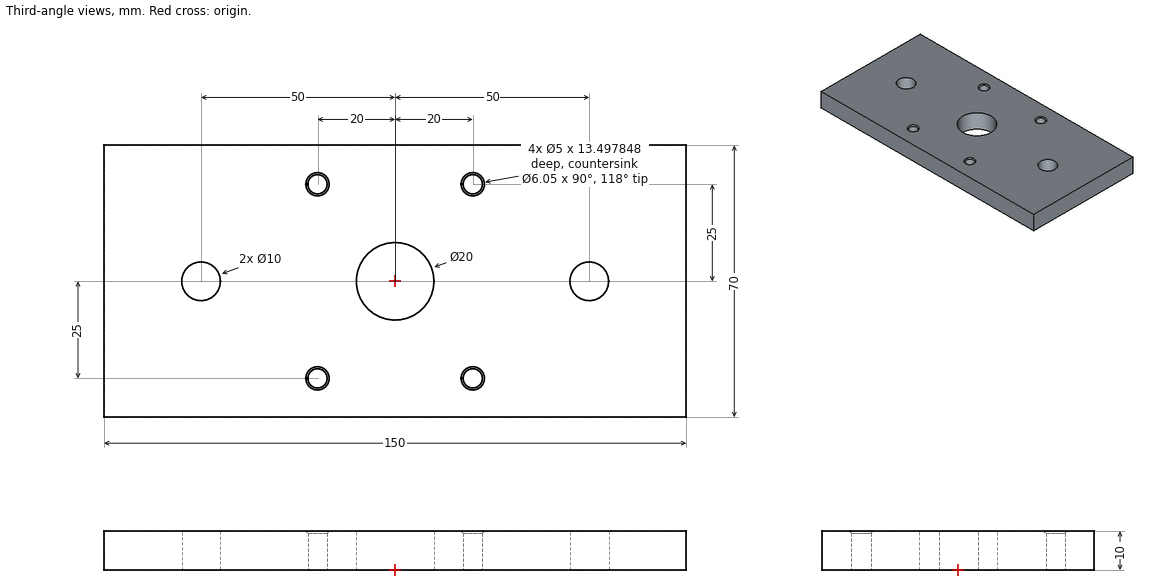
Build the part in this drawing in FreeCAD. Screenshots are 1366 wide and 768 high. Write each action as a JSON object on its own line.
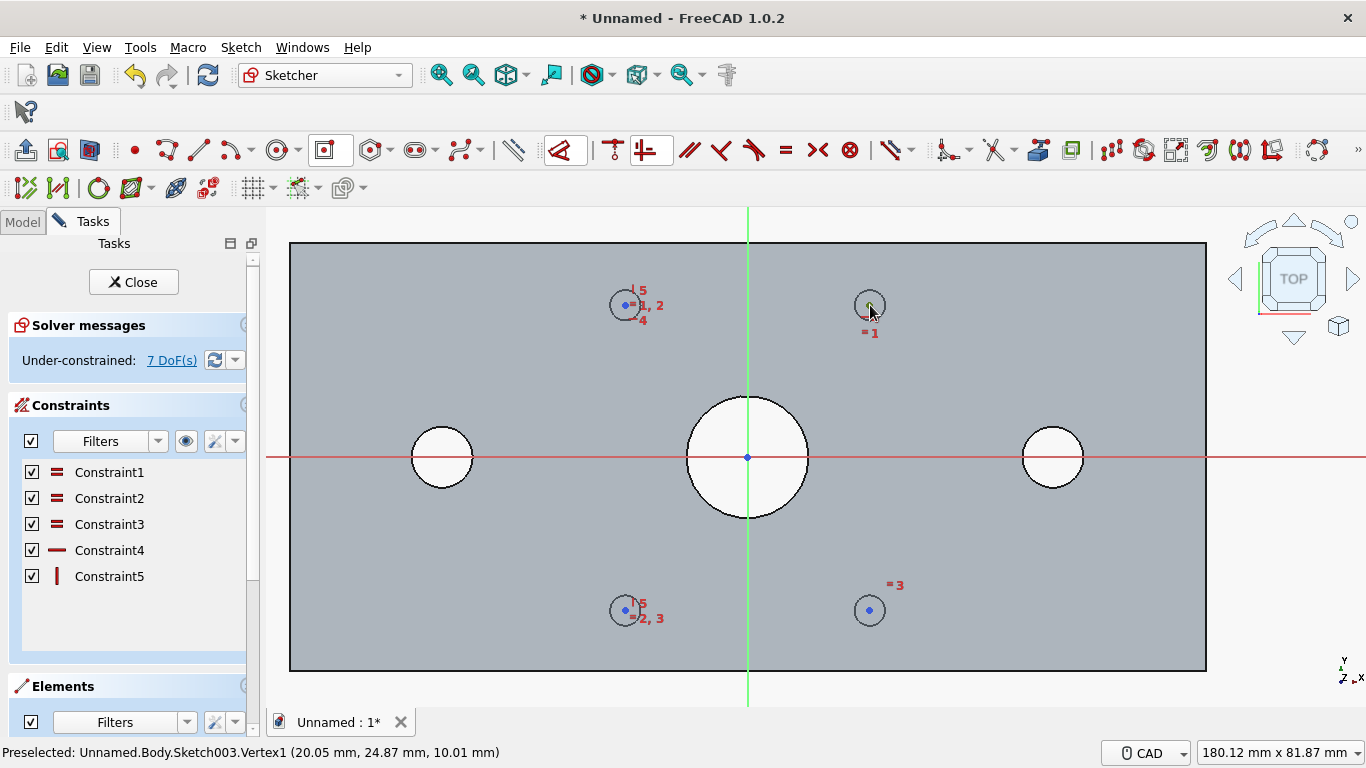
{"action": "left_click", "coordinate": [870, 611]}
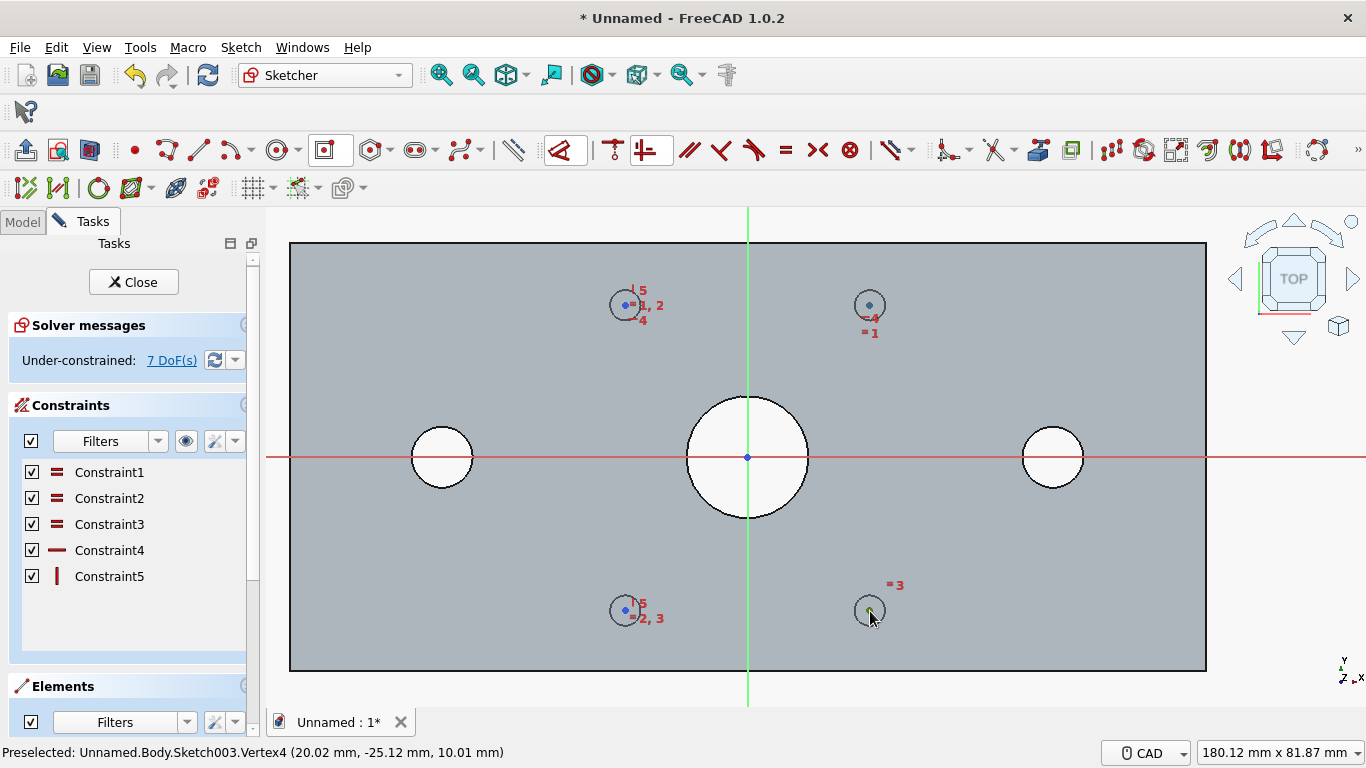
{"action": "left_click", "coordinate": [668, 150]}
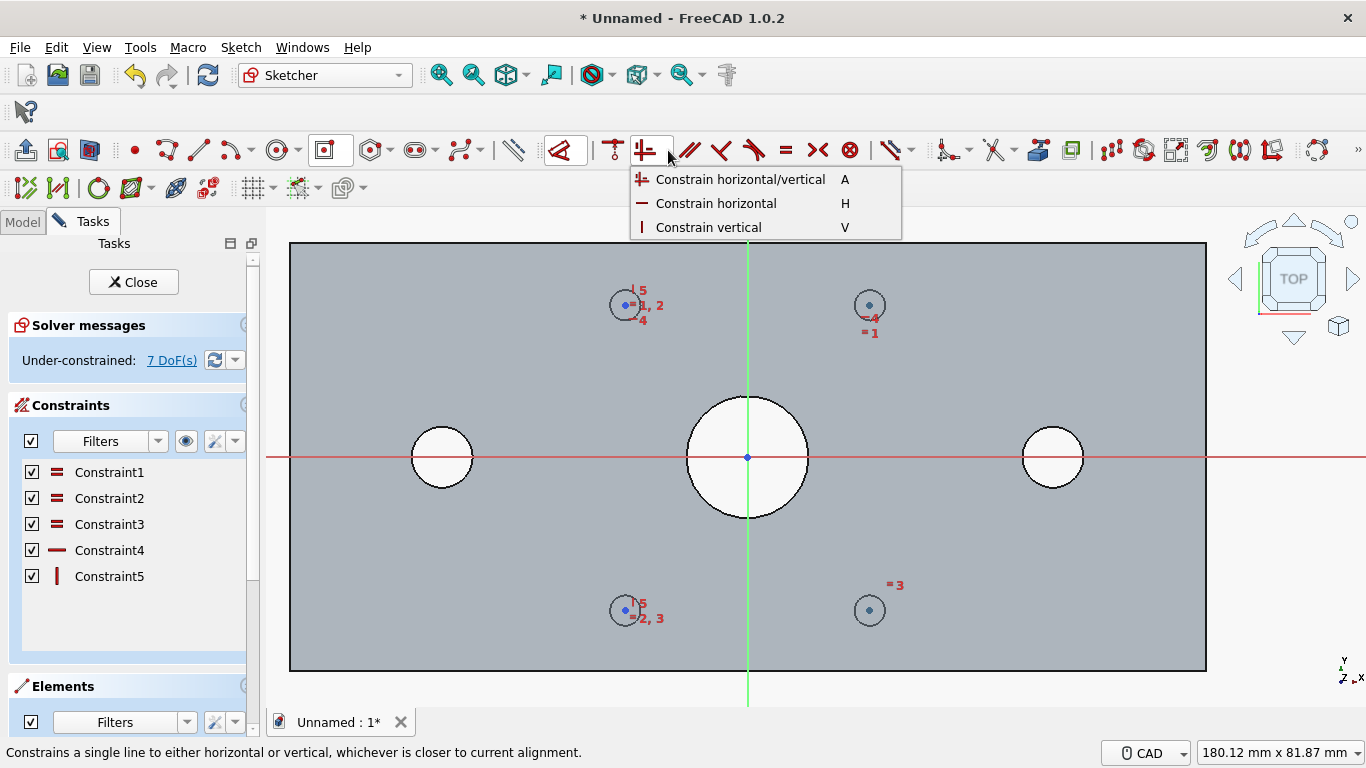
{"action": "left_click", "coordinate": [766, 227]}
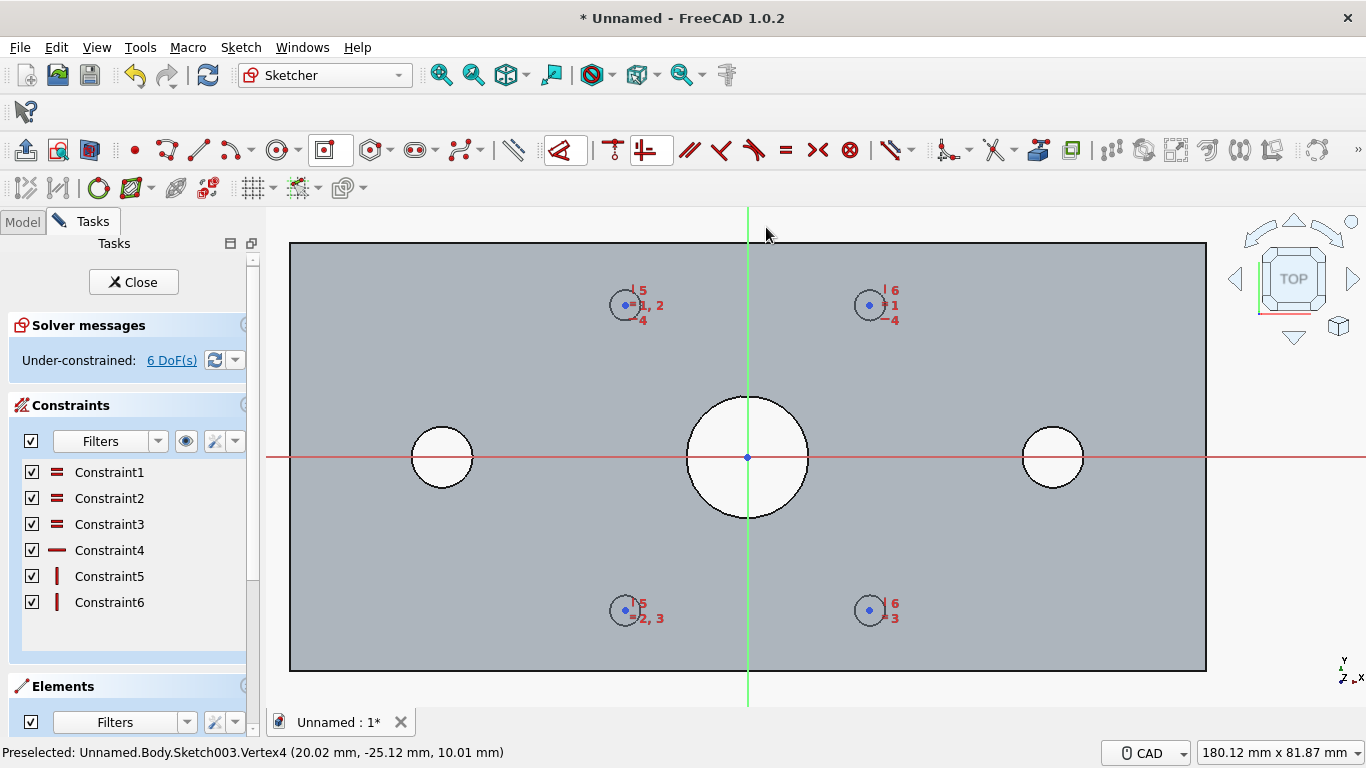
{"action": "left_click", "coordinate": [625, 611]}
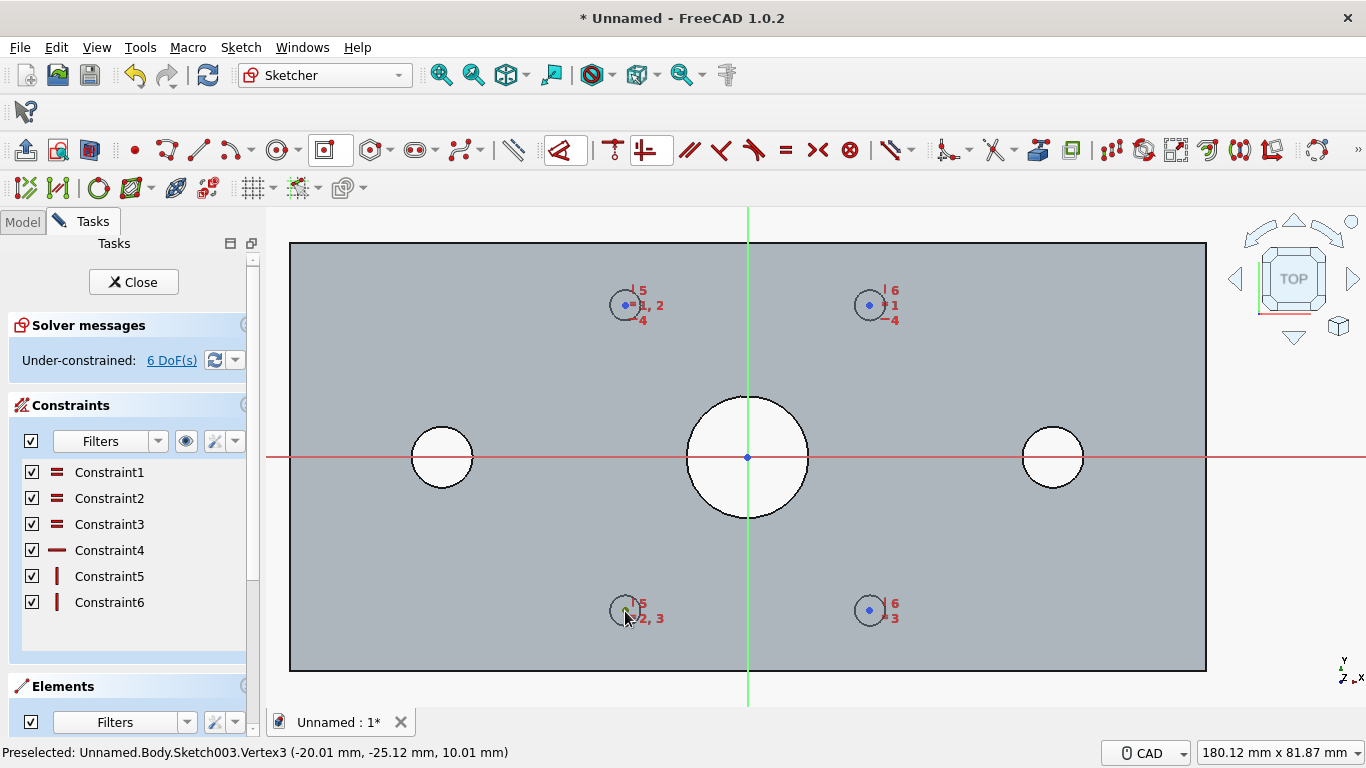
{"action": "left_click", "coordinate": [870, 611]}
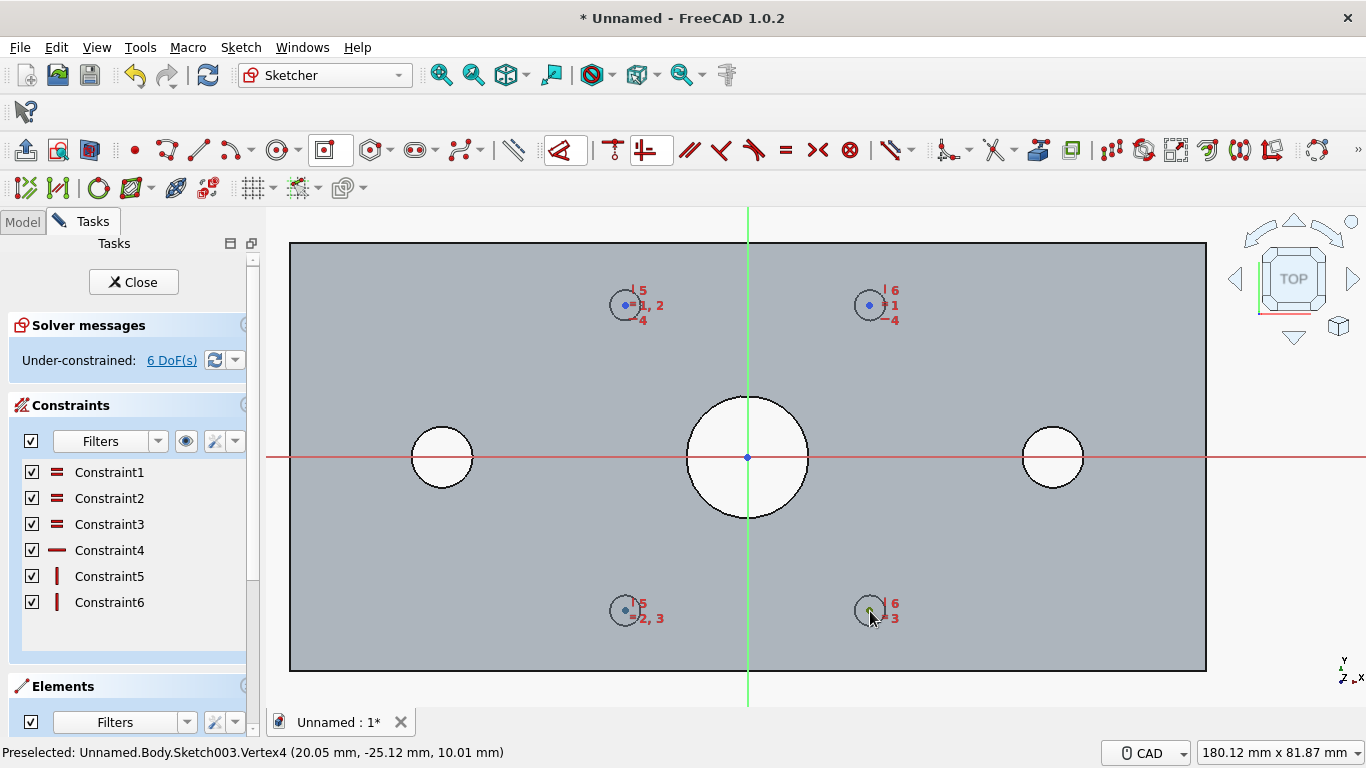
{"action": "left_click", "coordinate": [668, 150]}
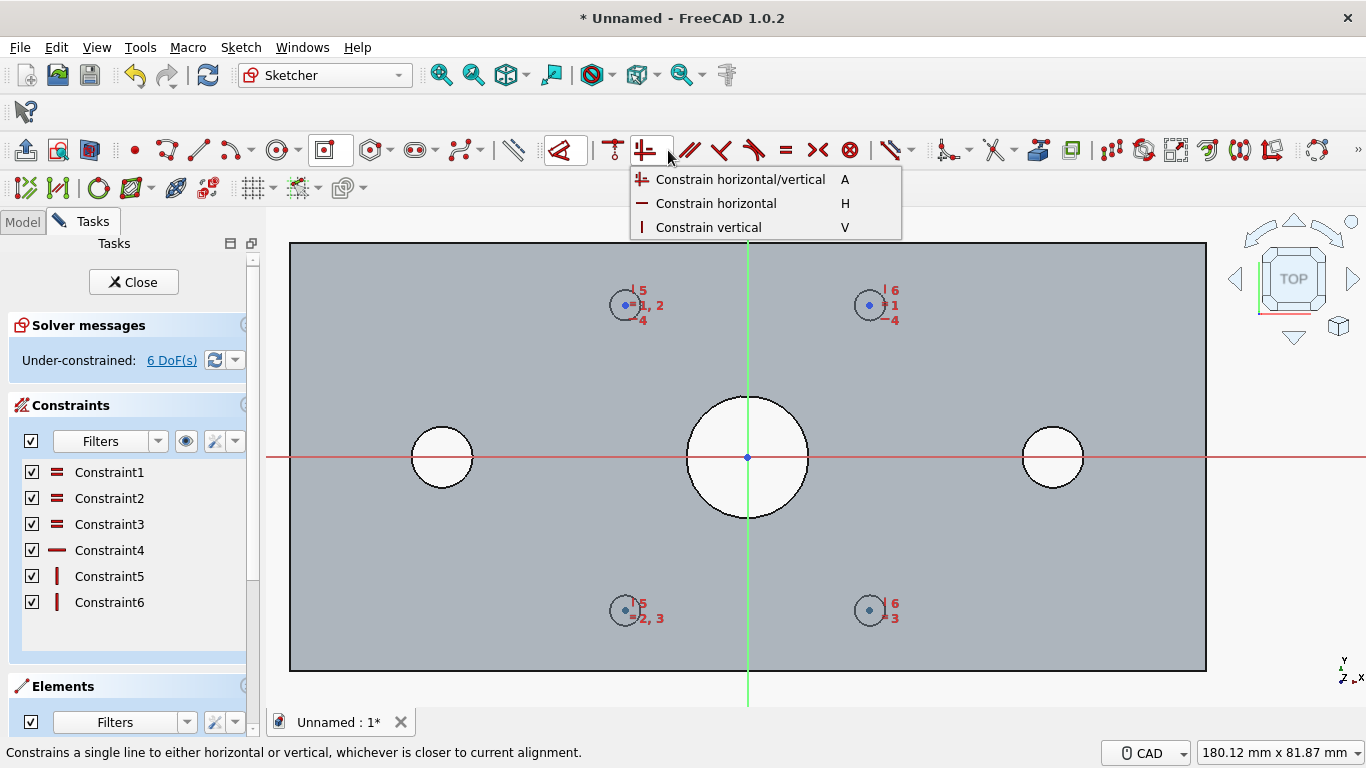
{"action": "left_click", "coordinate": [766, 203]}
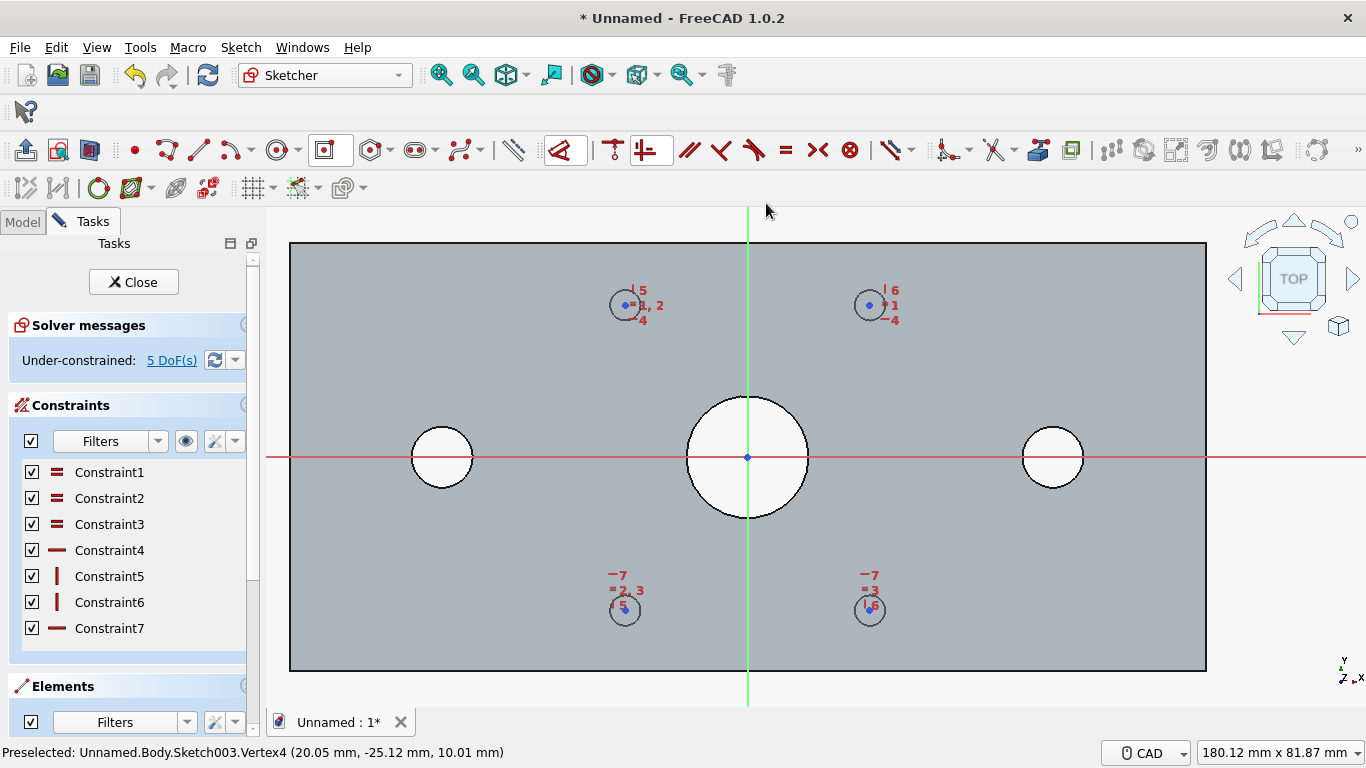
{"action": "scroll", "coordinate": [881, 295], "scroll_direction": "up", "scroll_amount": 2}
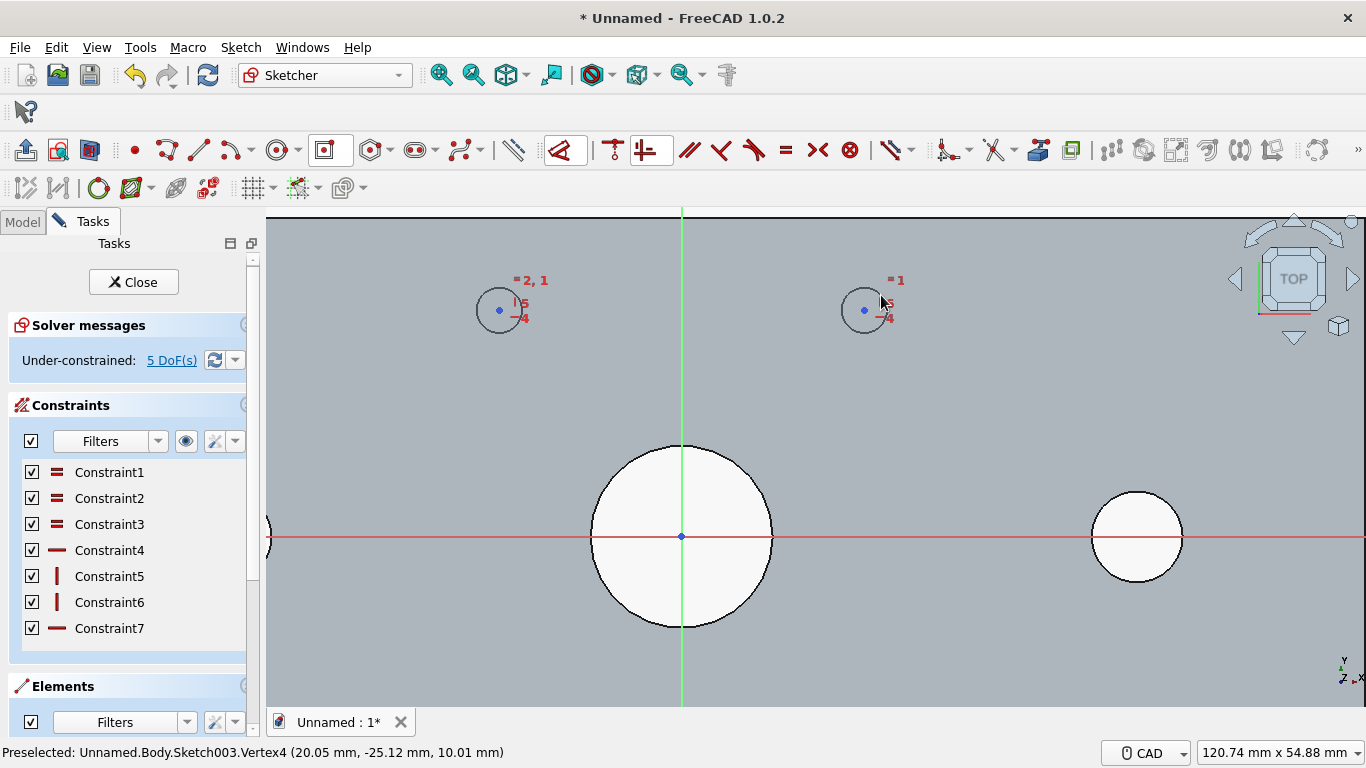
{"action": "left_click", "coordinate": [880, 294]}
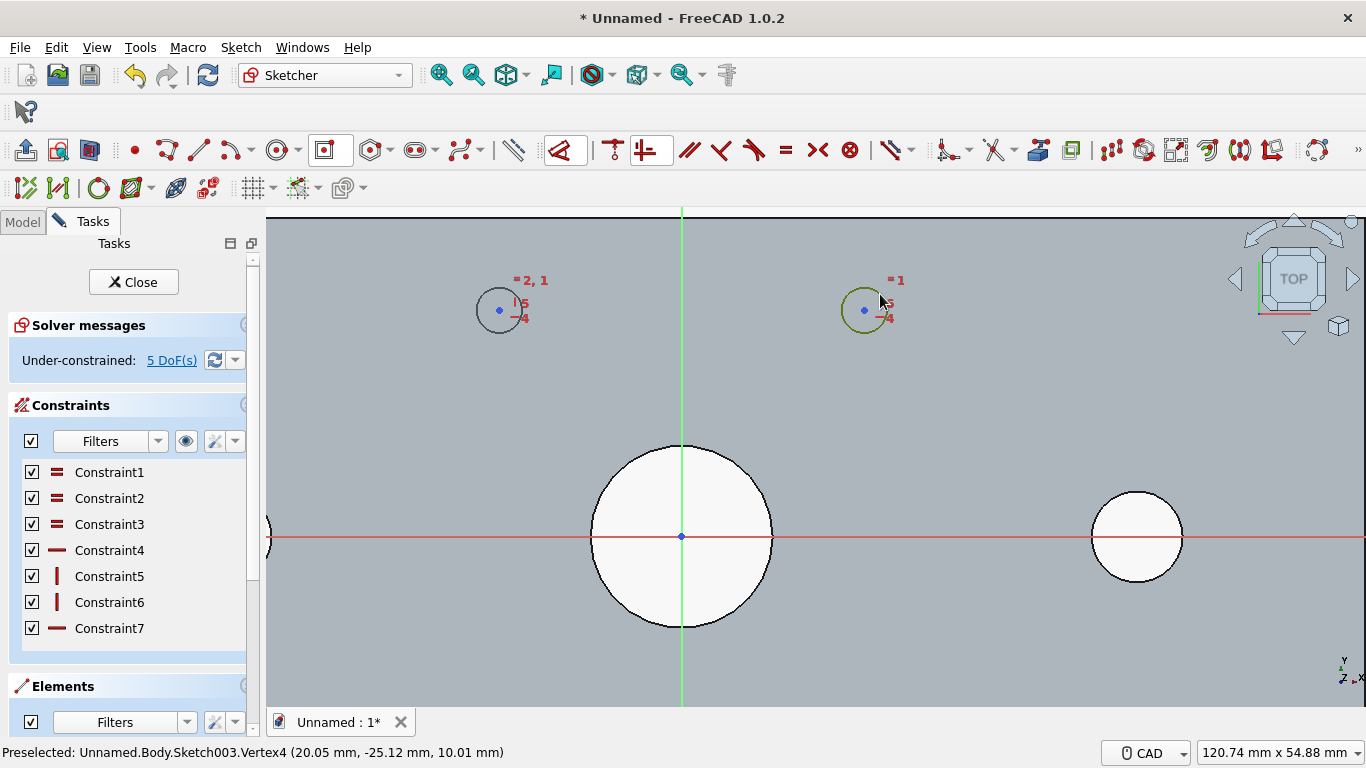
{"action": "left_click", "coordinate": [582, 150]}